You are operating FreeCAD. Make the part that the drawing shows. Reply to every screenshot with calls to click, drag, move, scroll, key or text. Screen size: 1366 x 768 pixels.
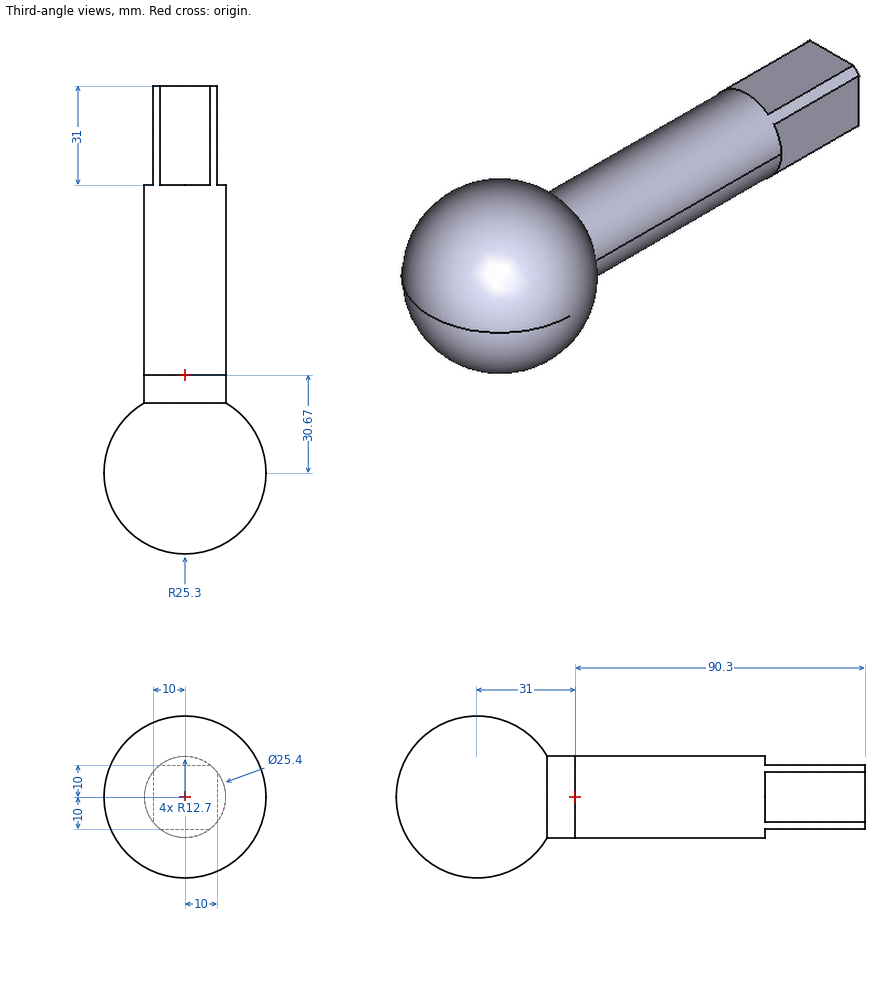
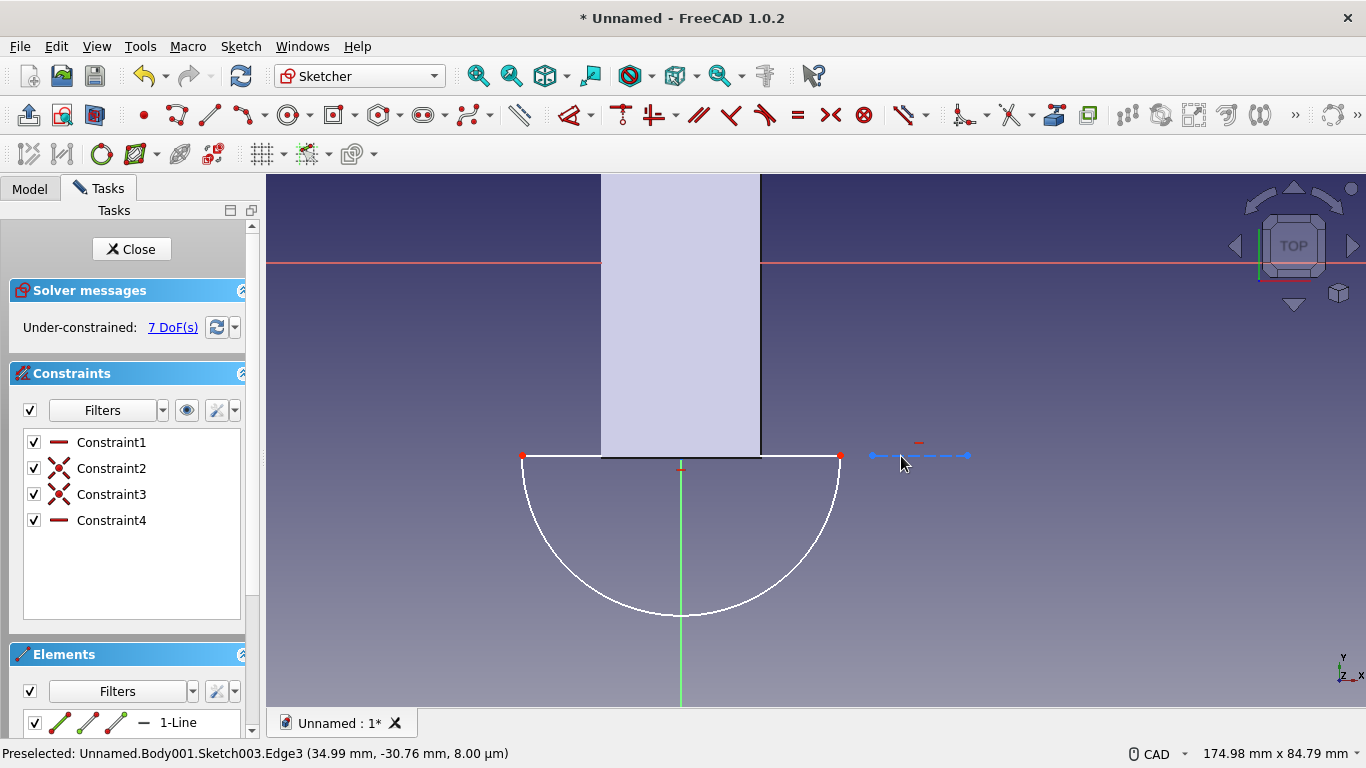
click(681, 457)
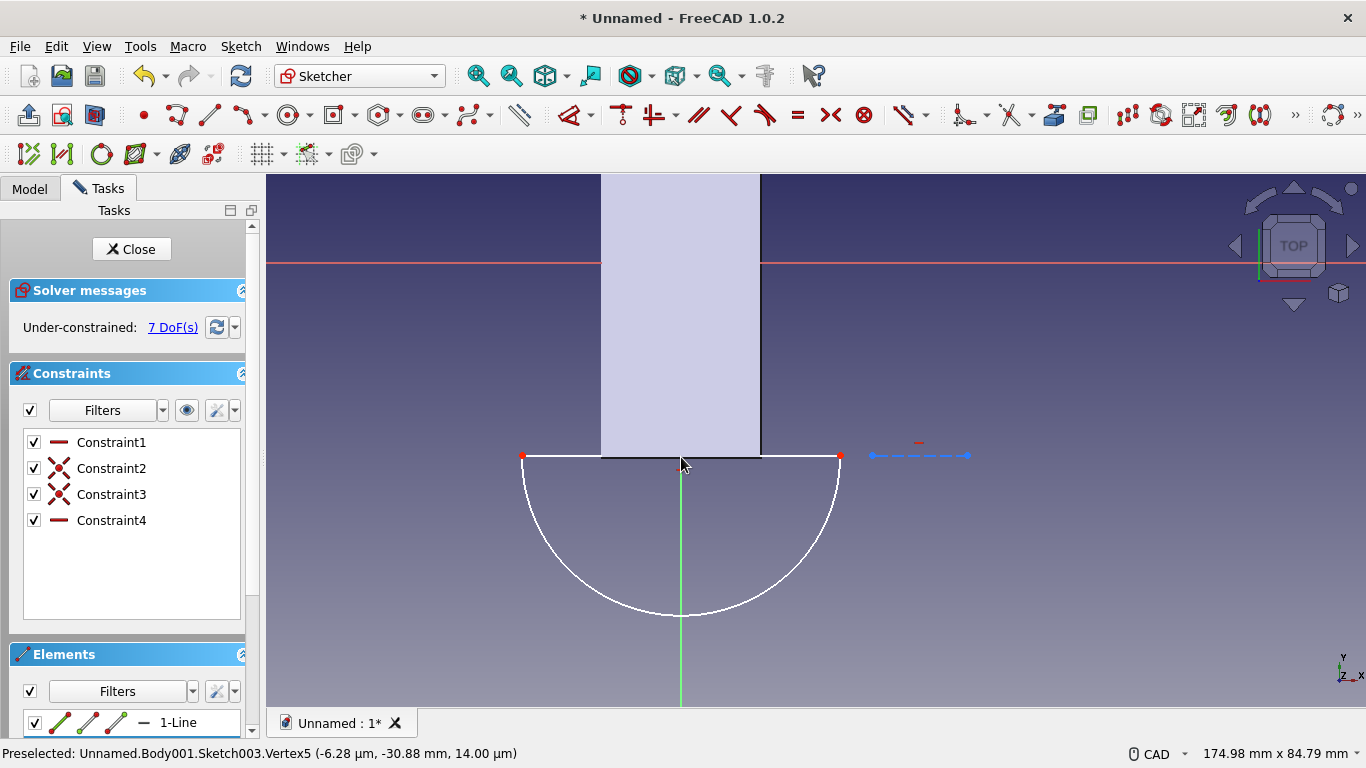
click(681, 577)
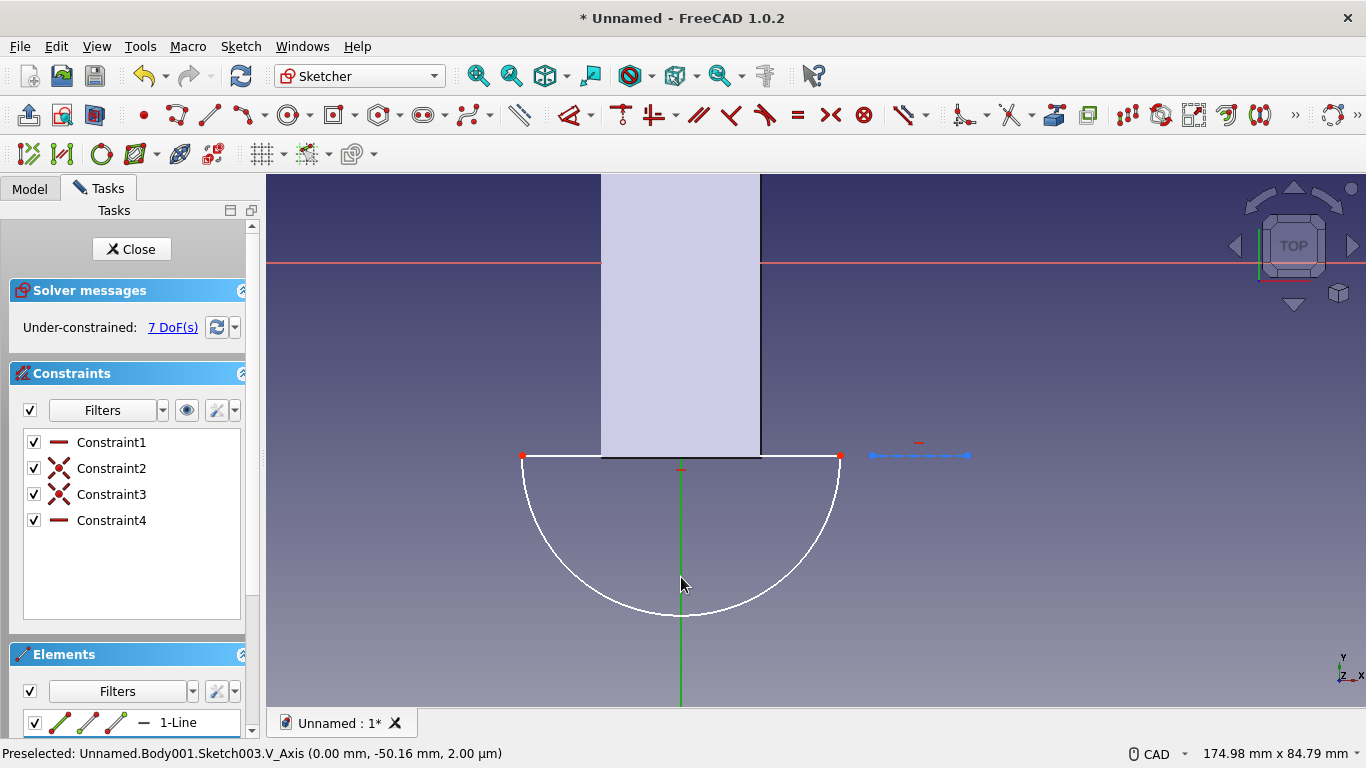
click(621, 116)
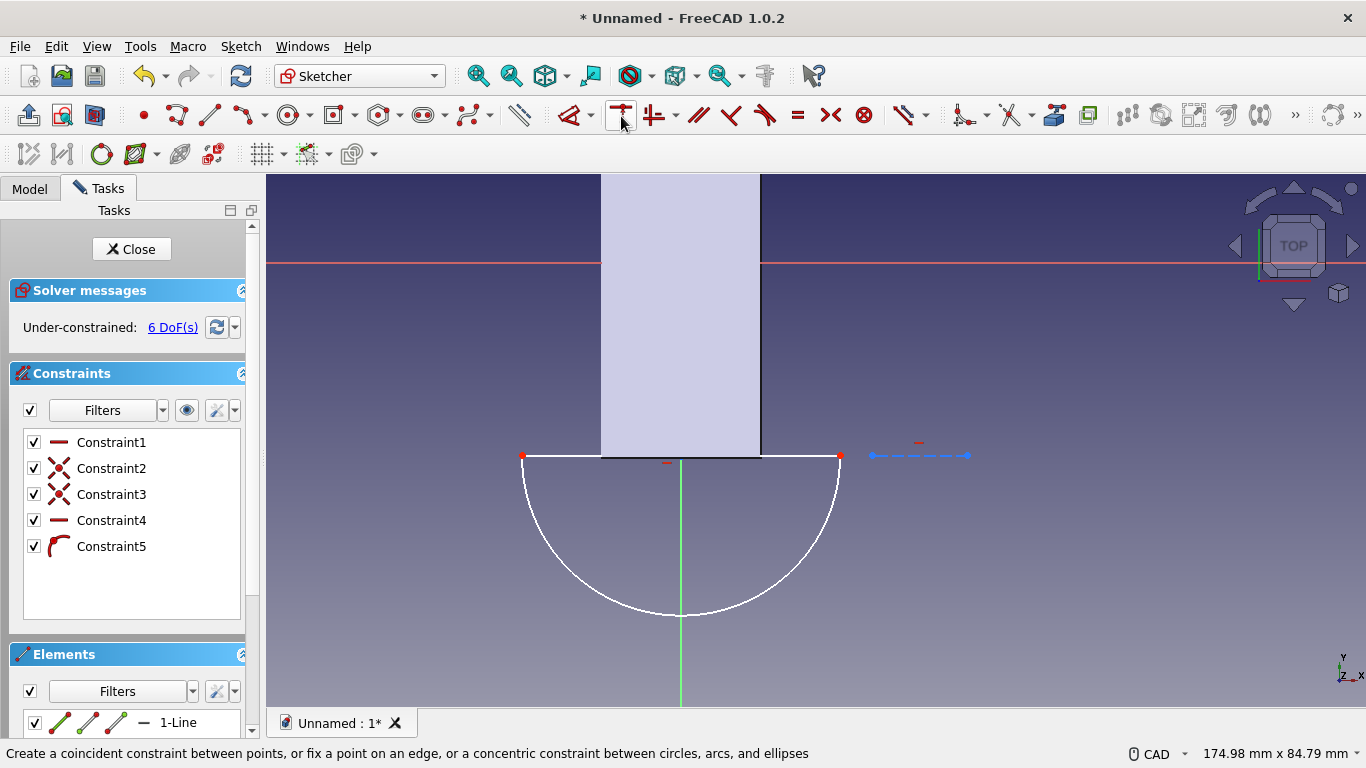
key(d)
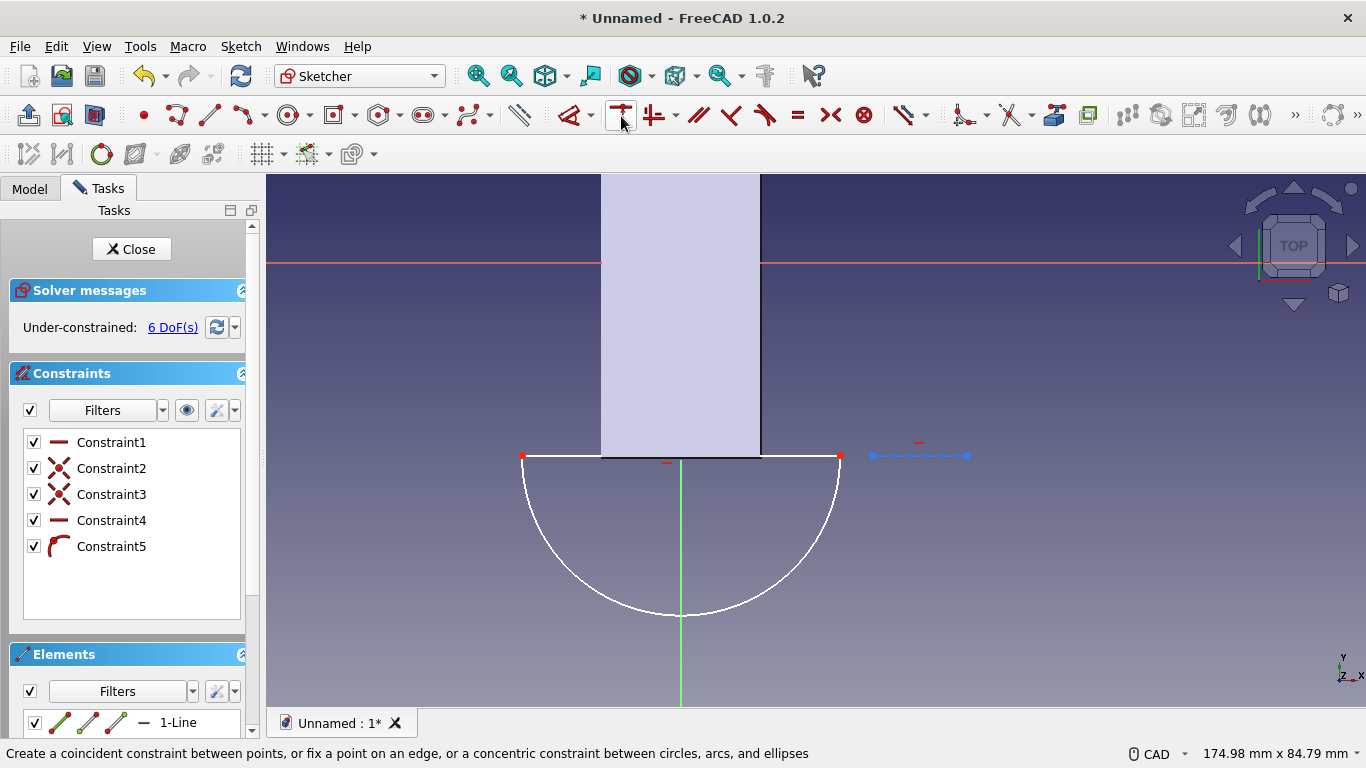
click(587, 585)
click(568, 611)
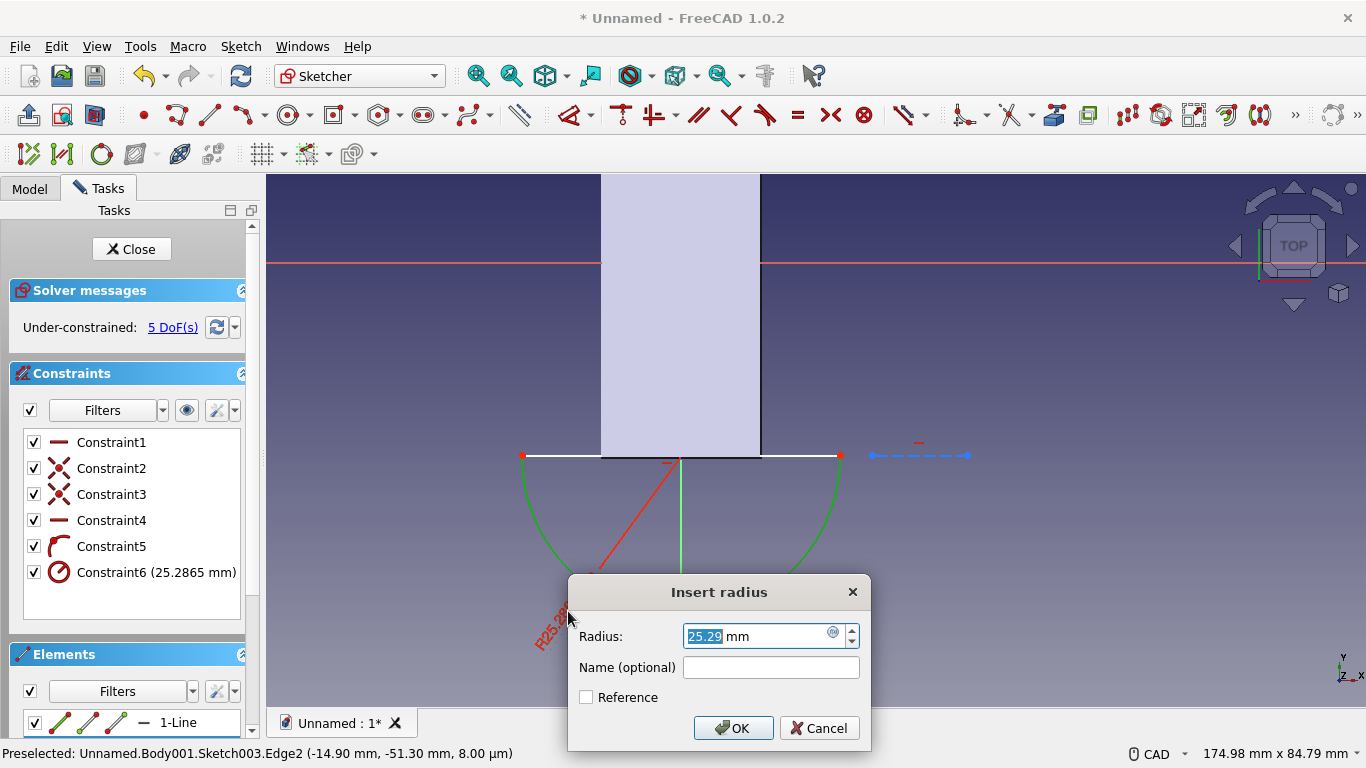
text(25.3)
key(Return)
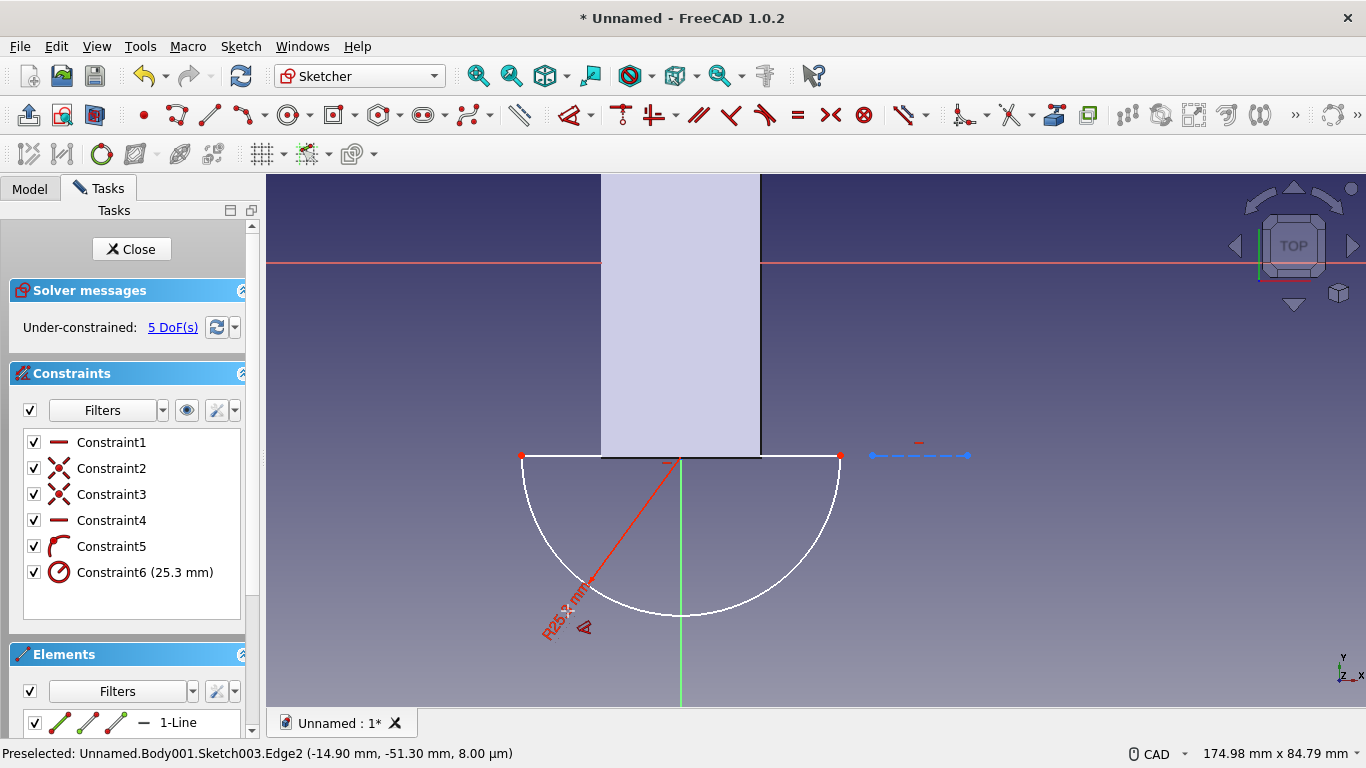
click(840, 456)
click(874, 359)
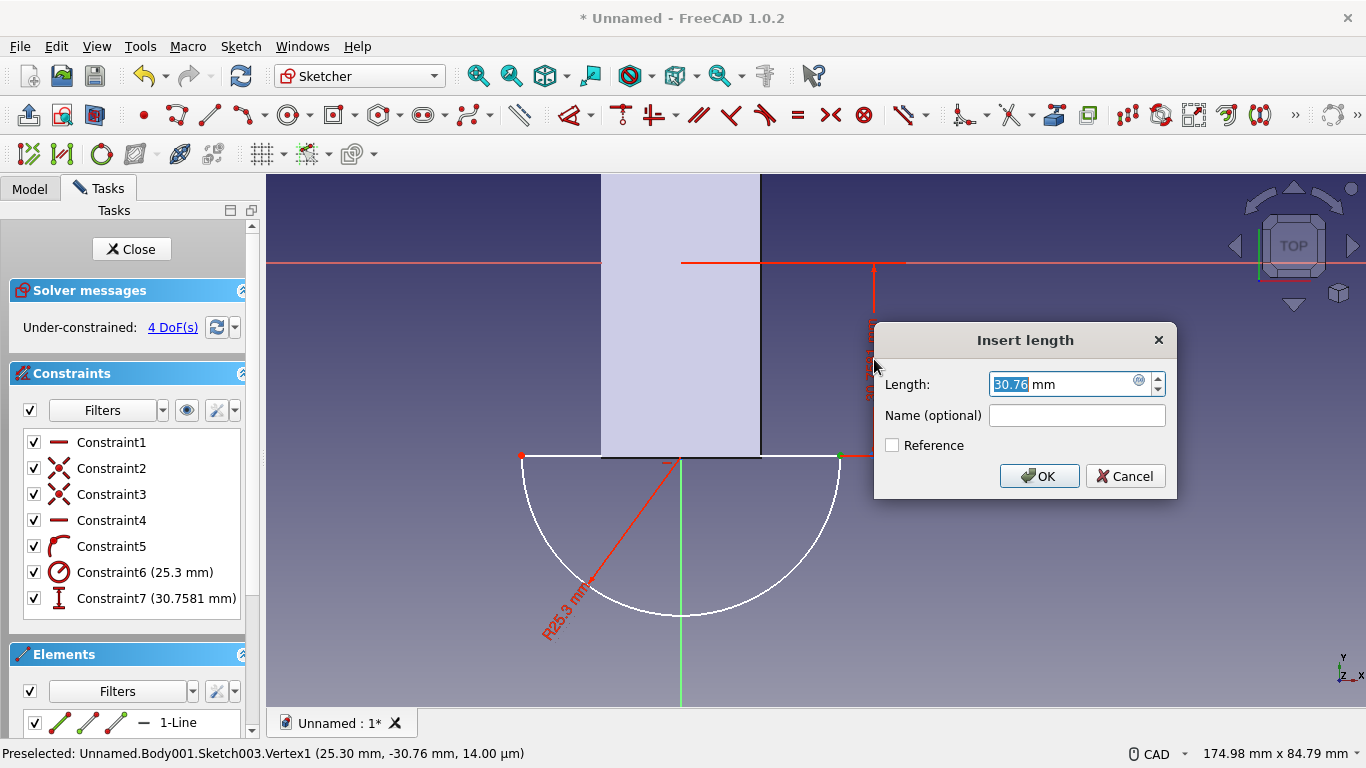
text(30.67)
key(Return)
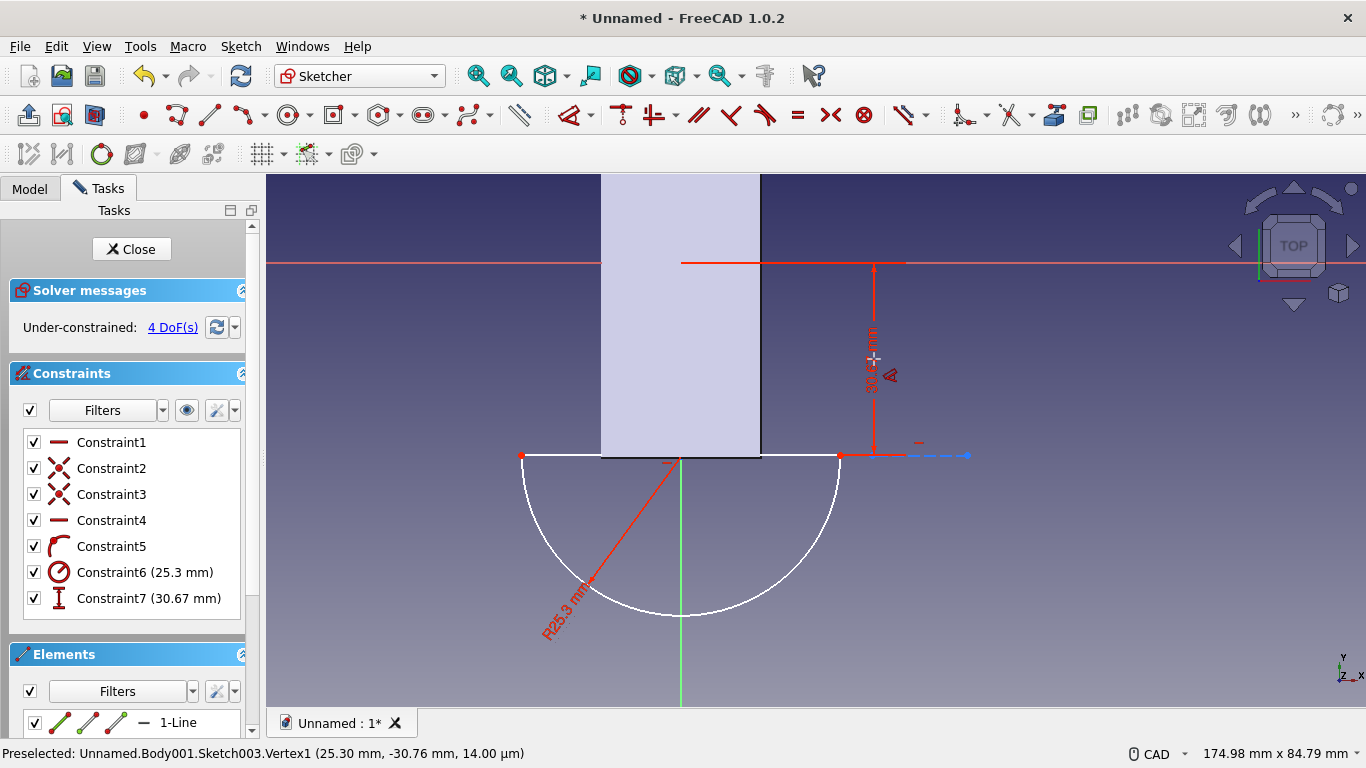
click(872, 456)
click(906, 315)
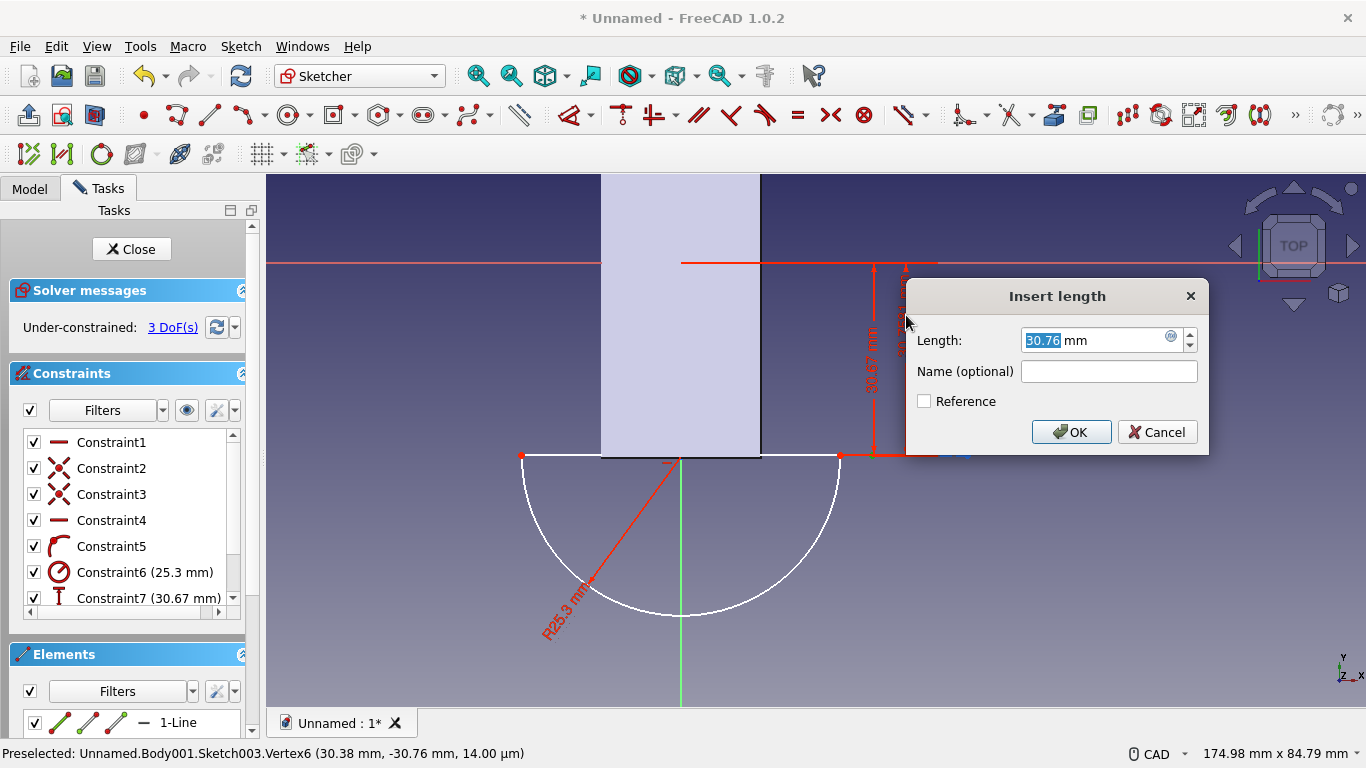
text(30.67)
key(Return)